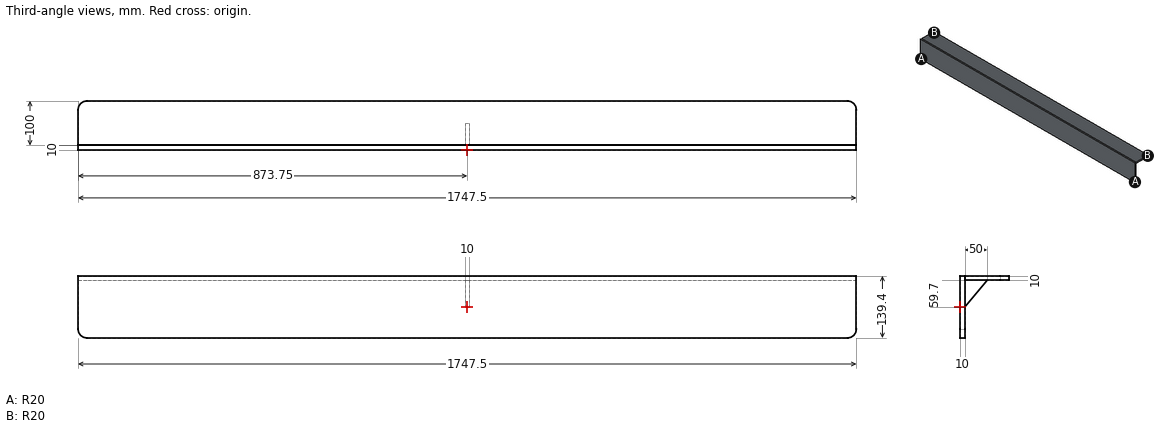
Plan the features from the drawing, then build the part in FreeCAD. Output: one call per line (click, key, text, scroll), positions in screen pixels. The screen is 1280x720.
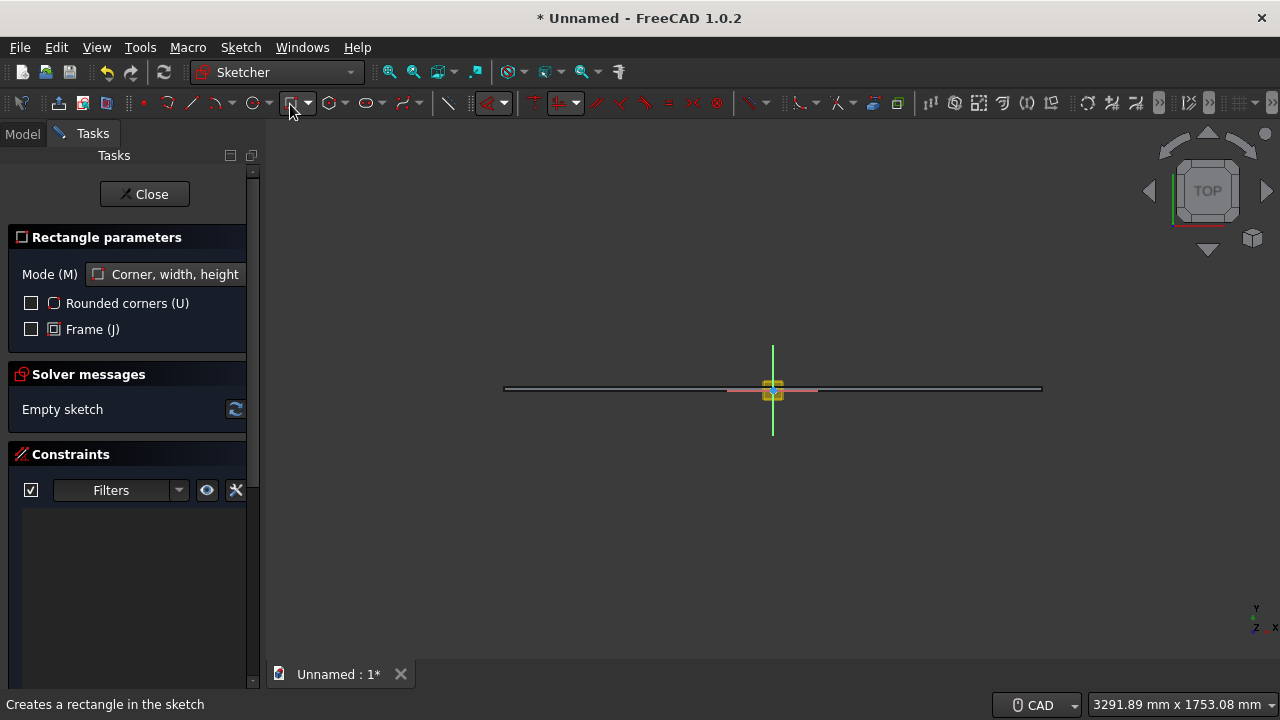
click(504, 357)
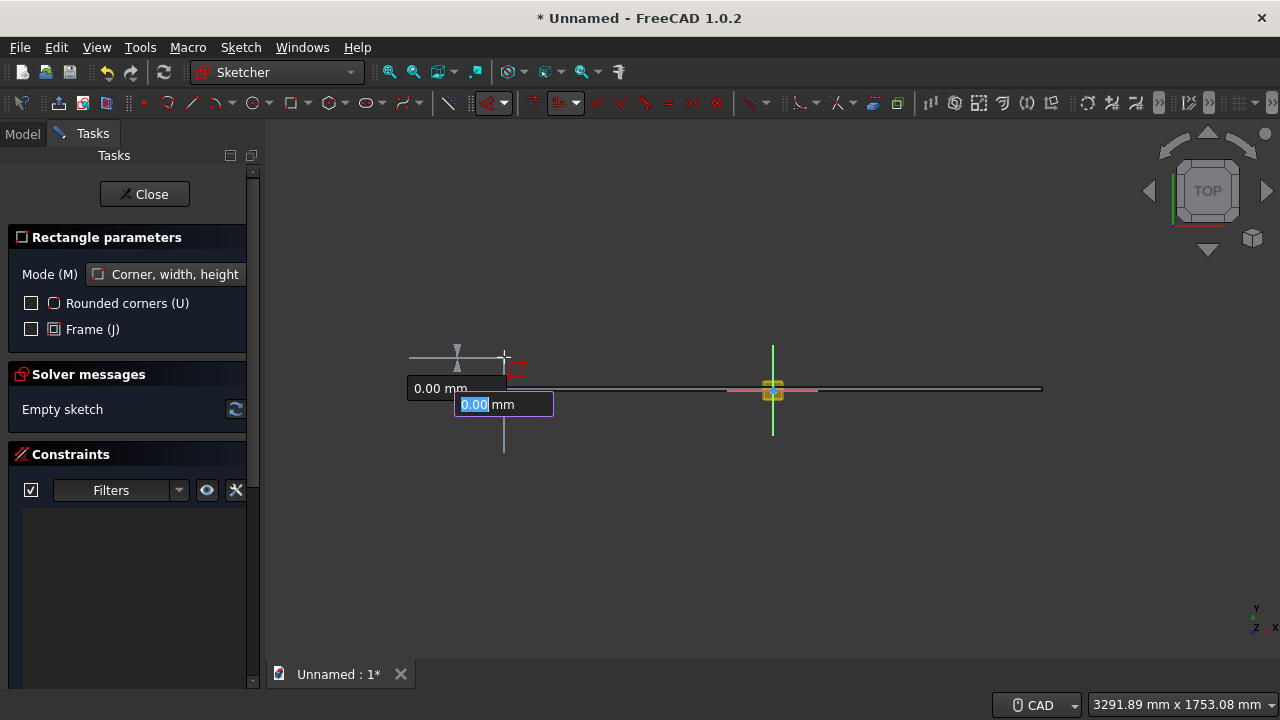
scroll(1042, 387, up, 9)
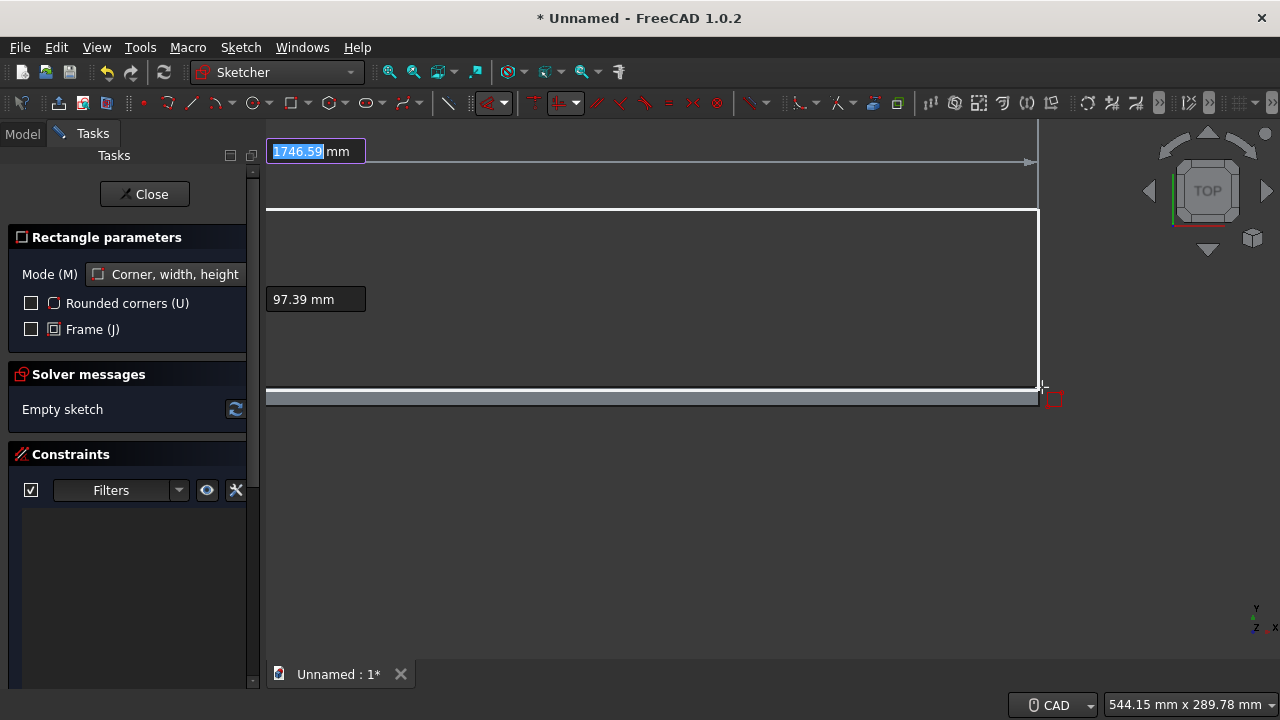
click(1039, 387)
key(Escape)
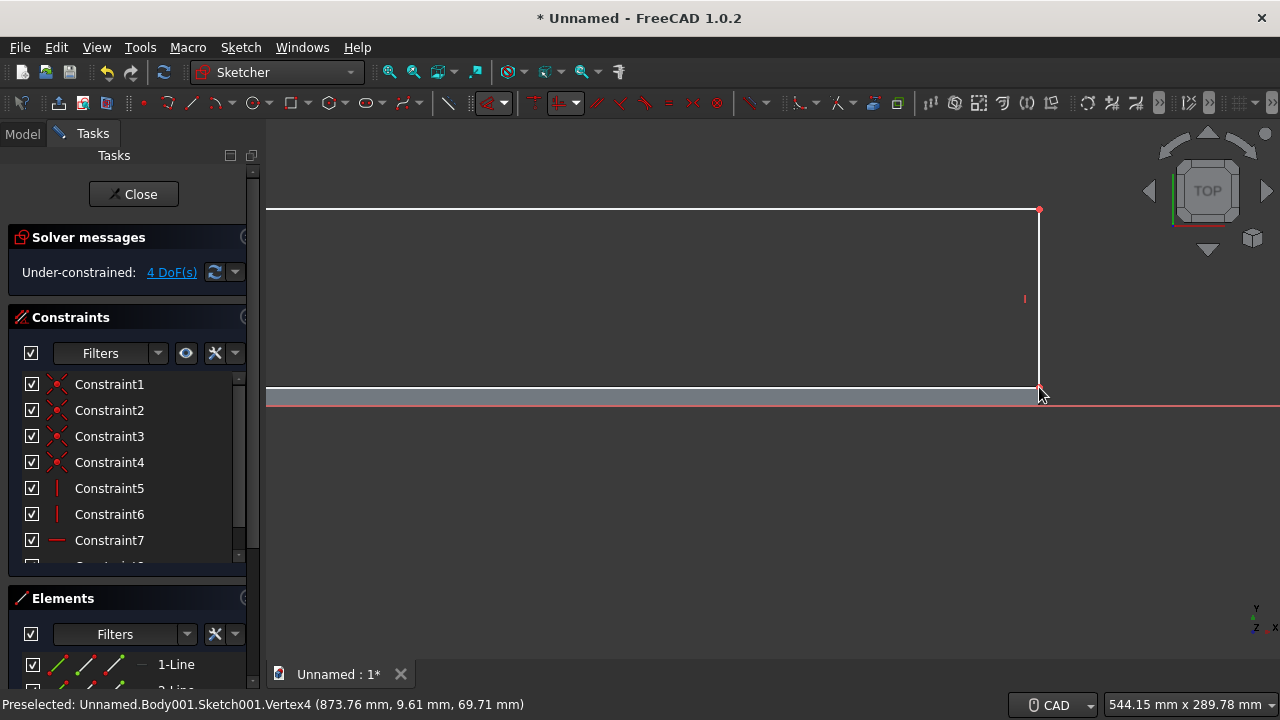
scroll(961, 406, down, 9)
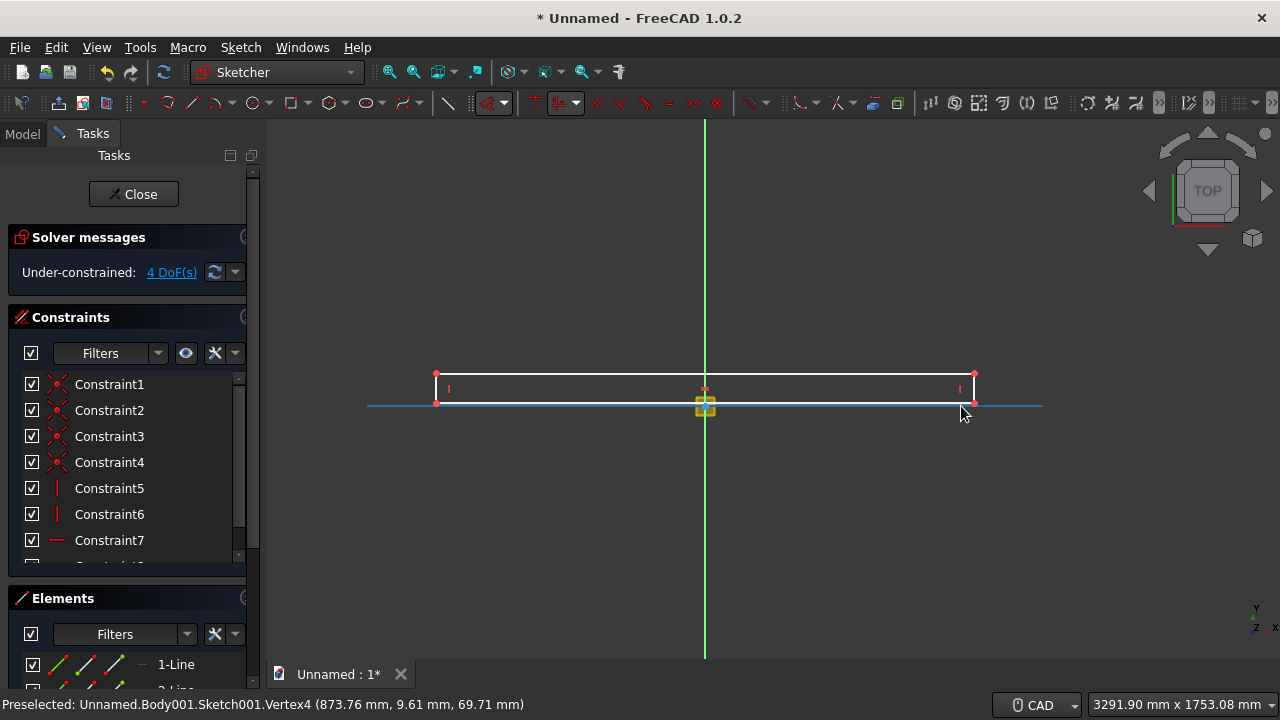
scroll(436, 383, up, 3)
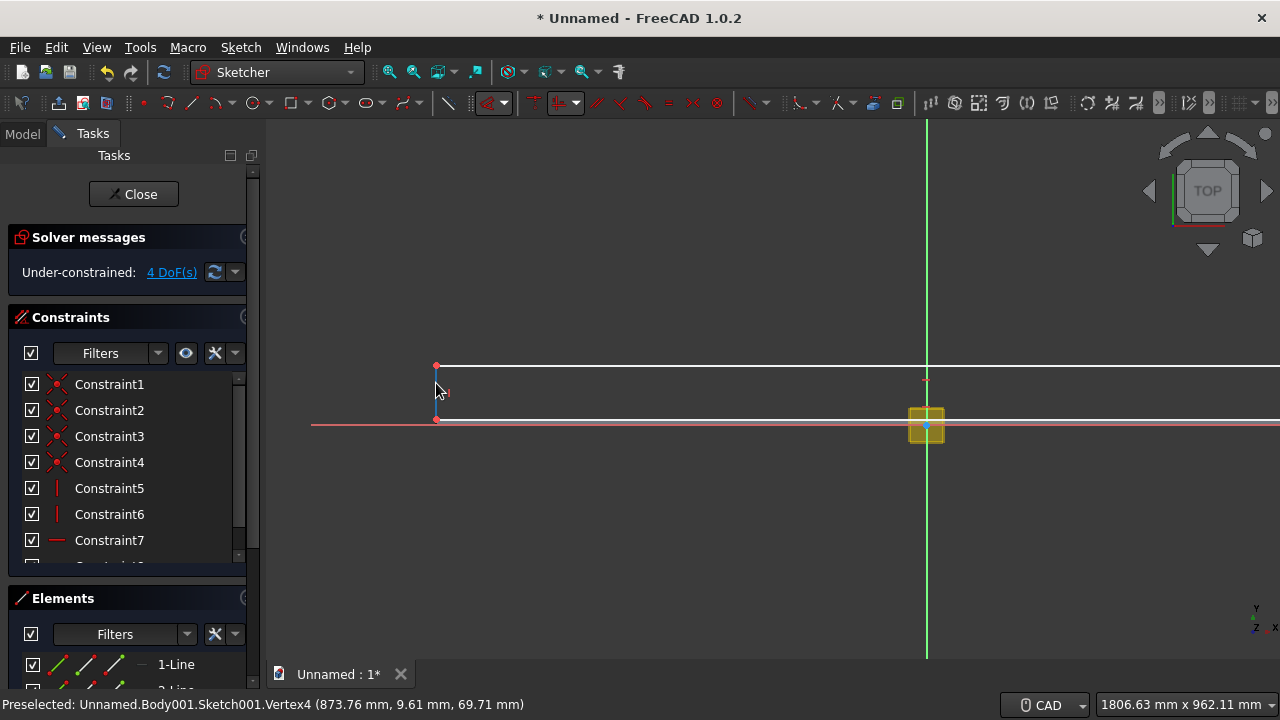
click(436, 382)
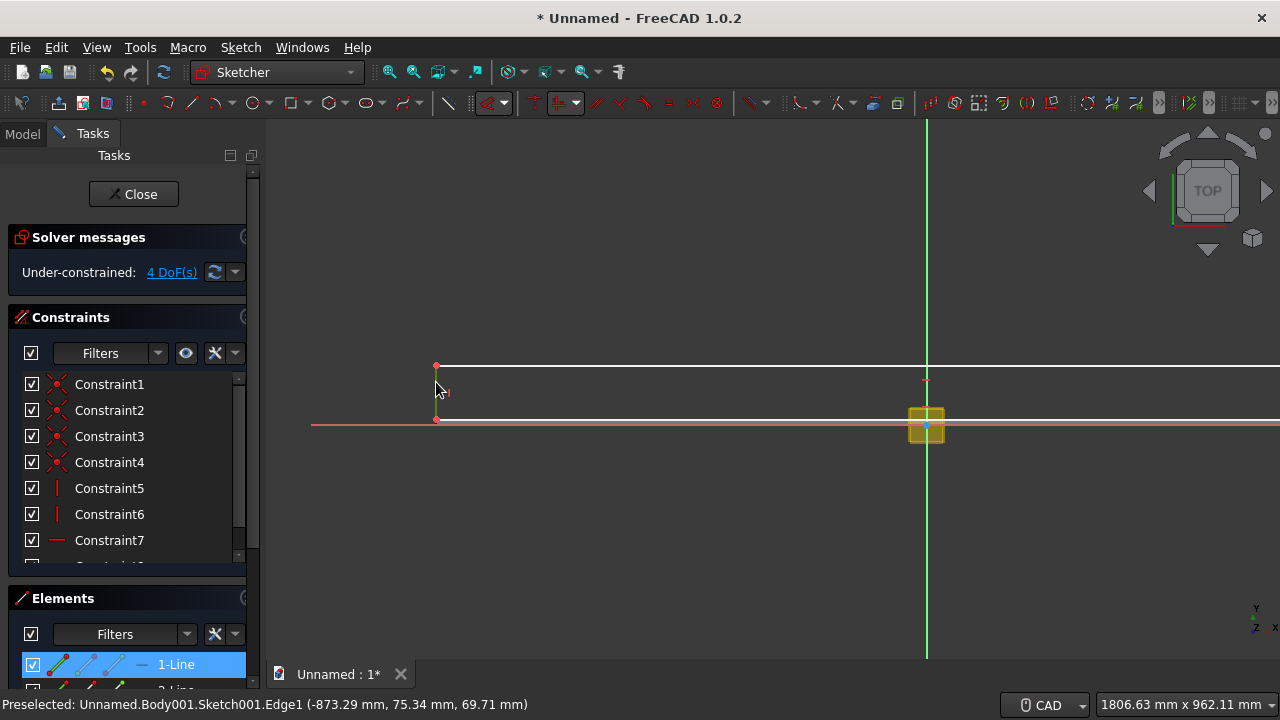
click(506, 104)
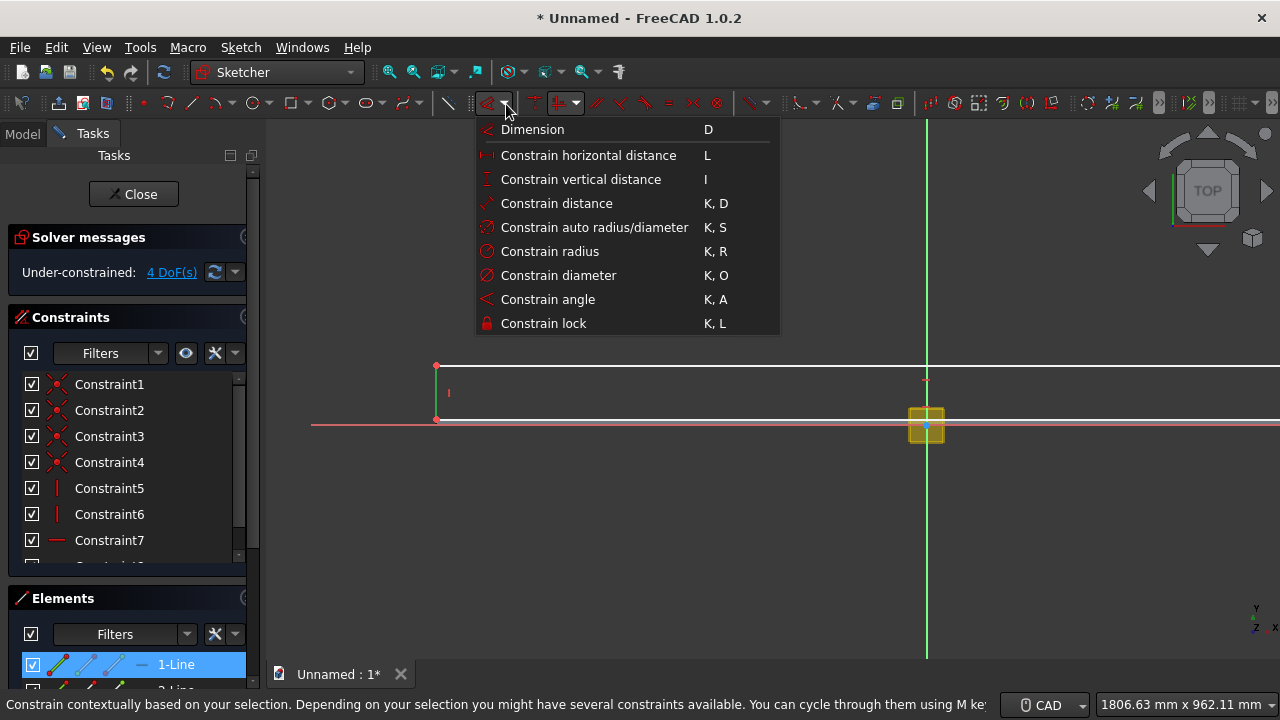
click(628, 179)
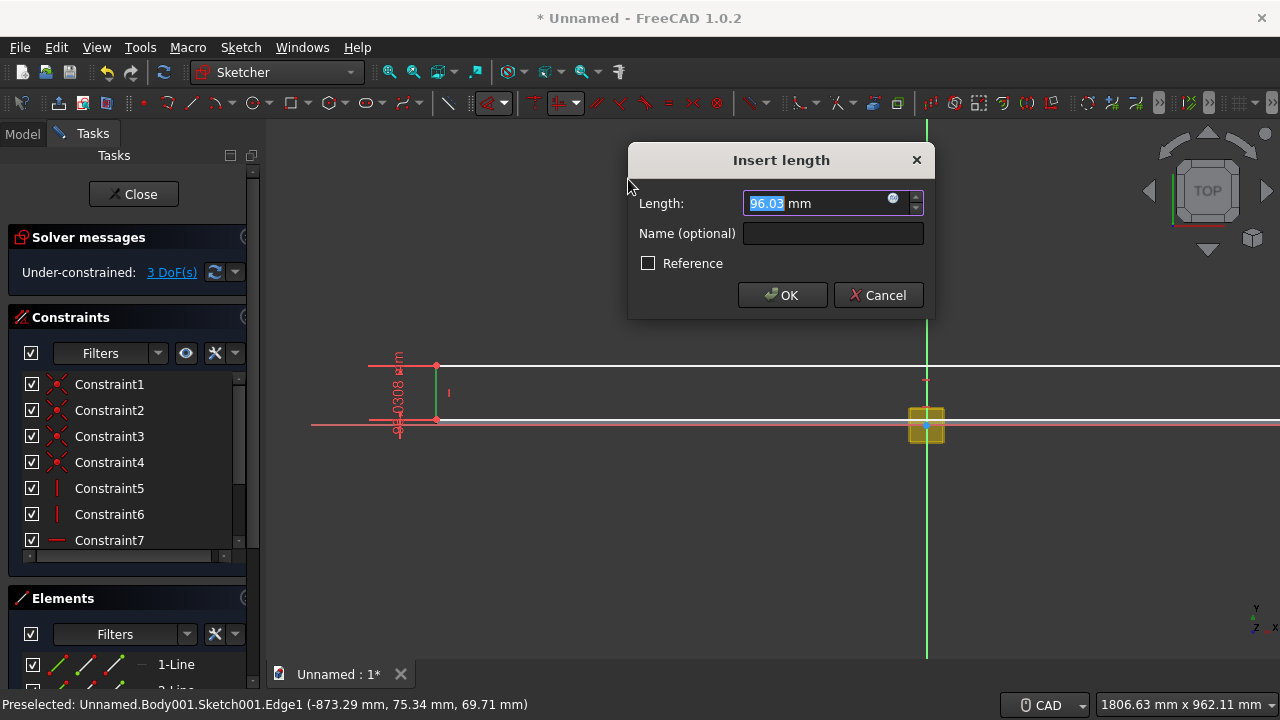
text(100)
key(Return)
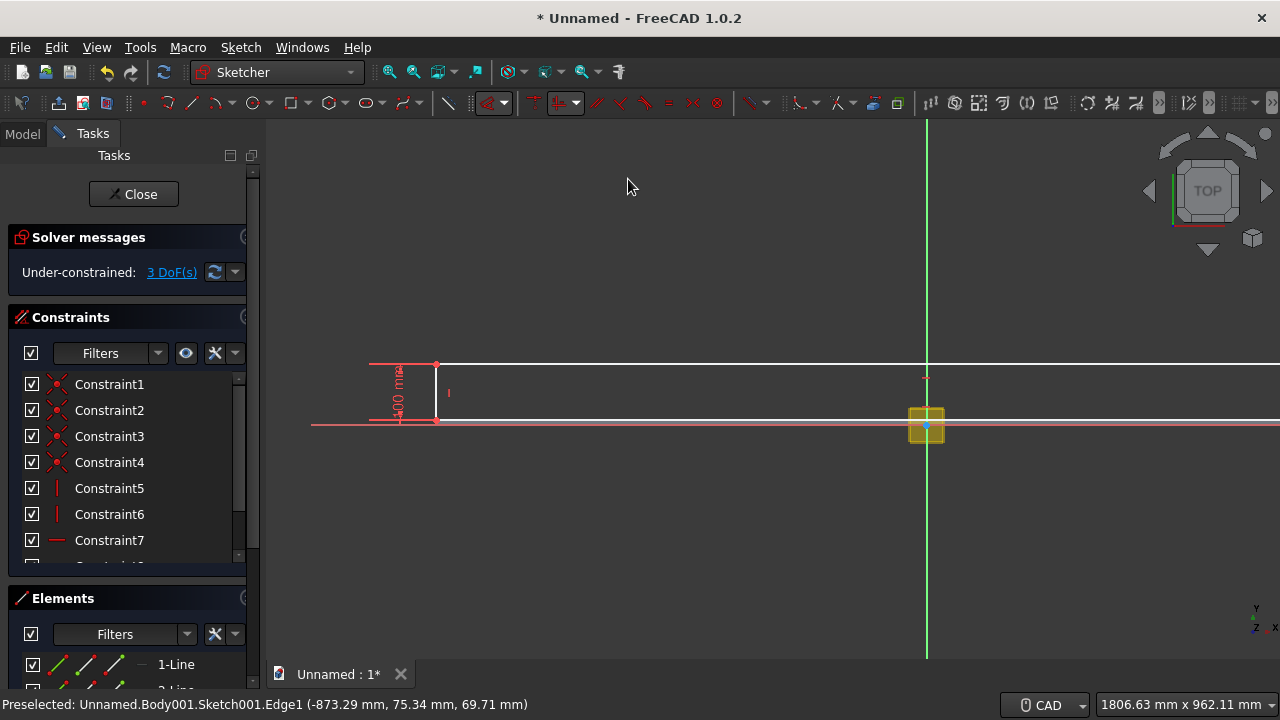
scroll(436, 420, up, 10)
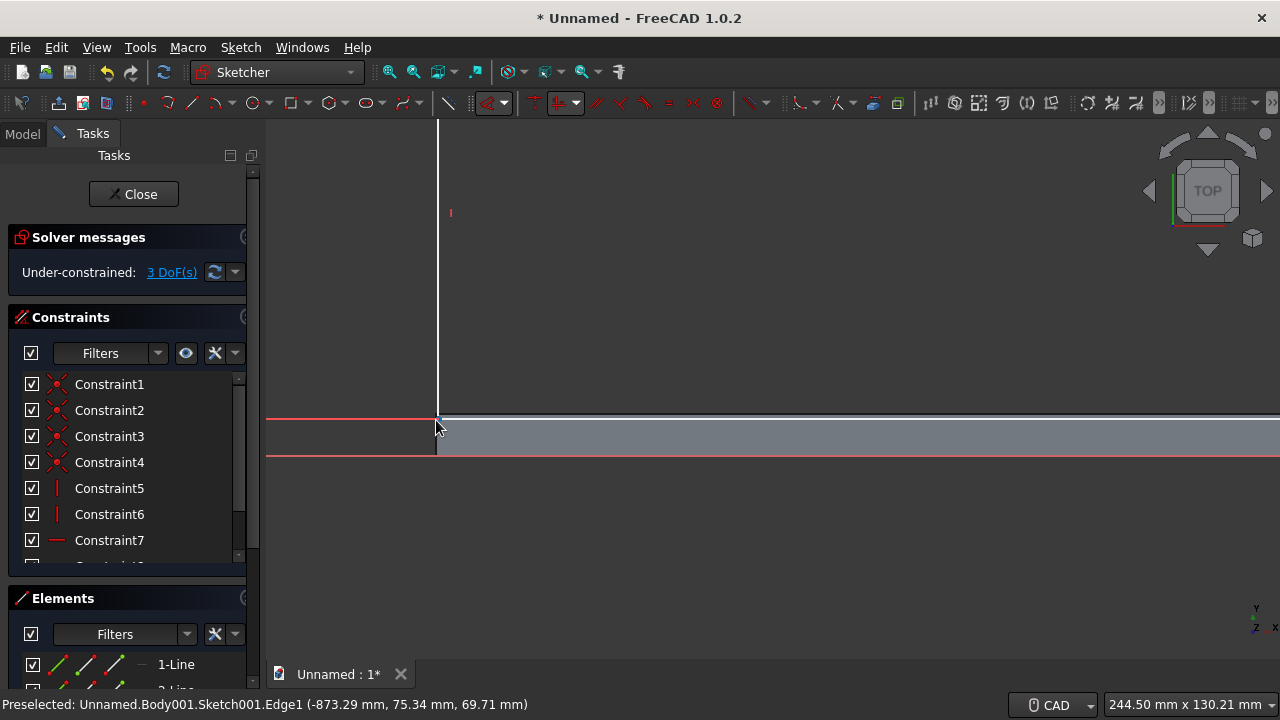
click(438, 419)